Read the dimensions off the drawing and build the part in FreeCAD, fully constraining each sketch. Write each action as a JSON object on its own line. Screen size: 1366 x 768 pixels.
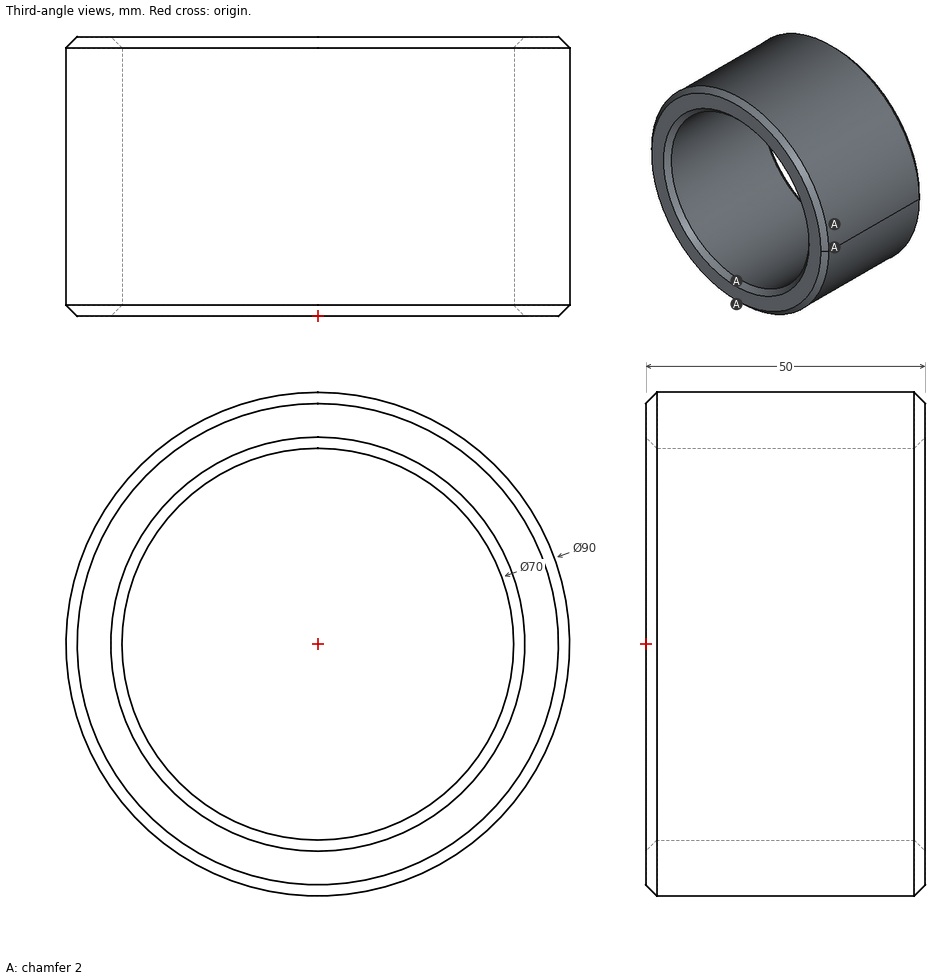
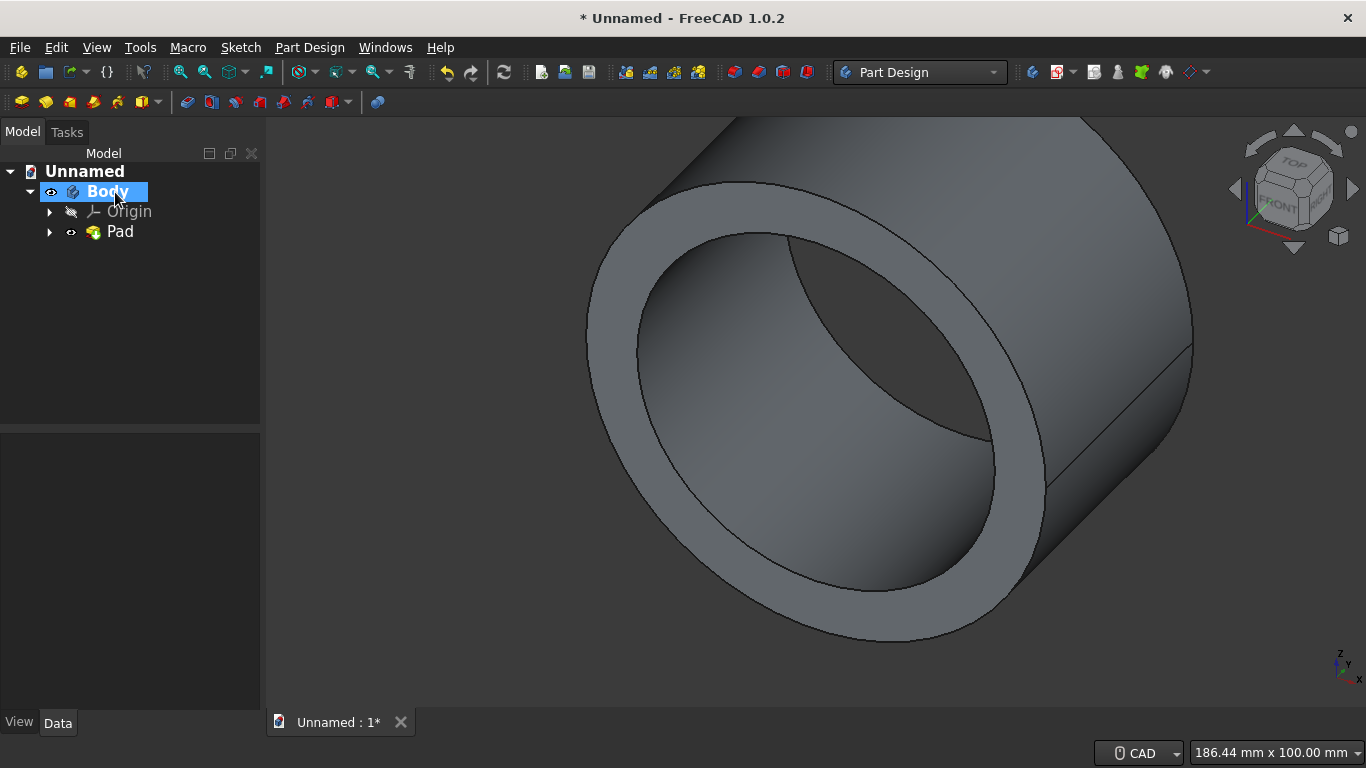
{"action": "left_click", "coordinate": [182, 72]}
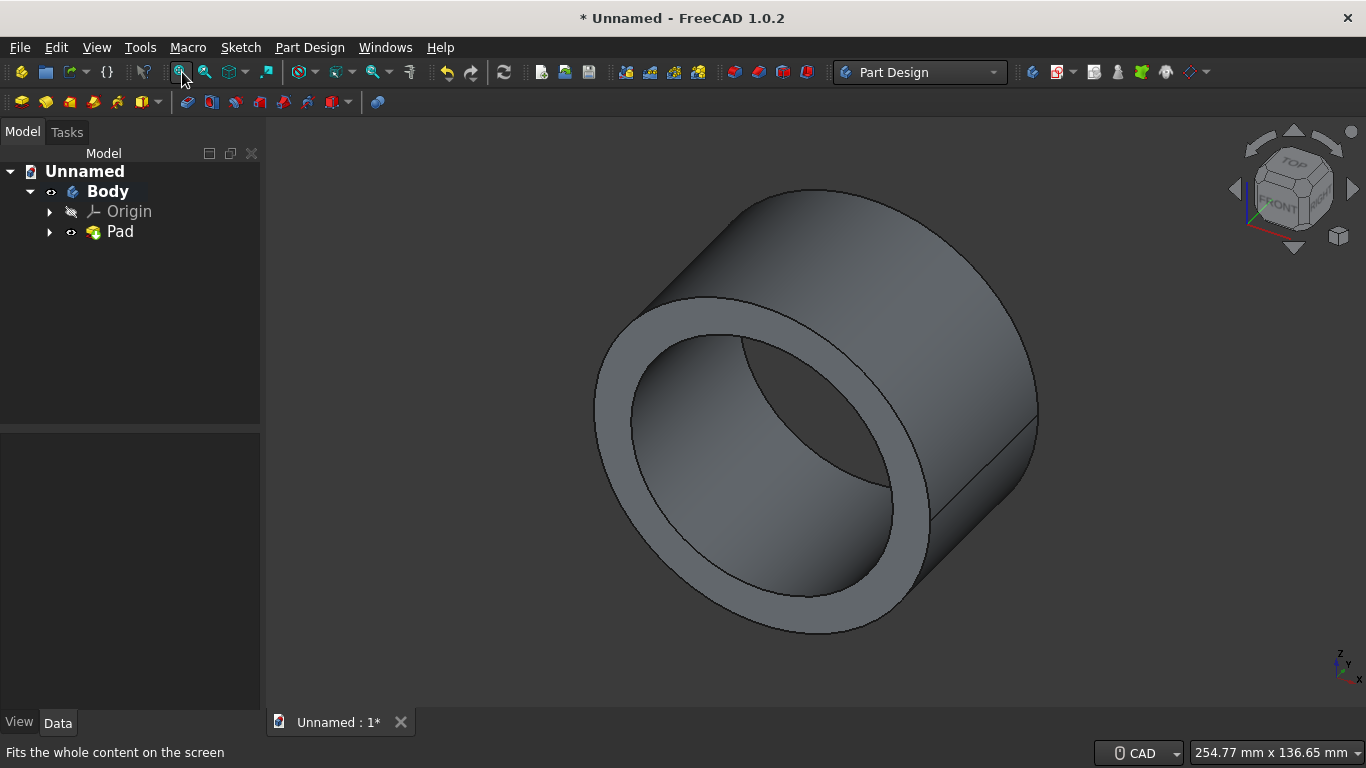
{"action": "left_click", "coordinate": [626, 326]}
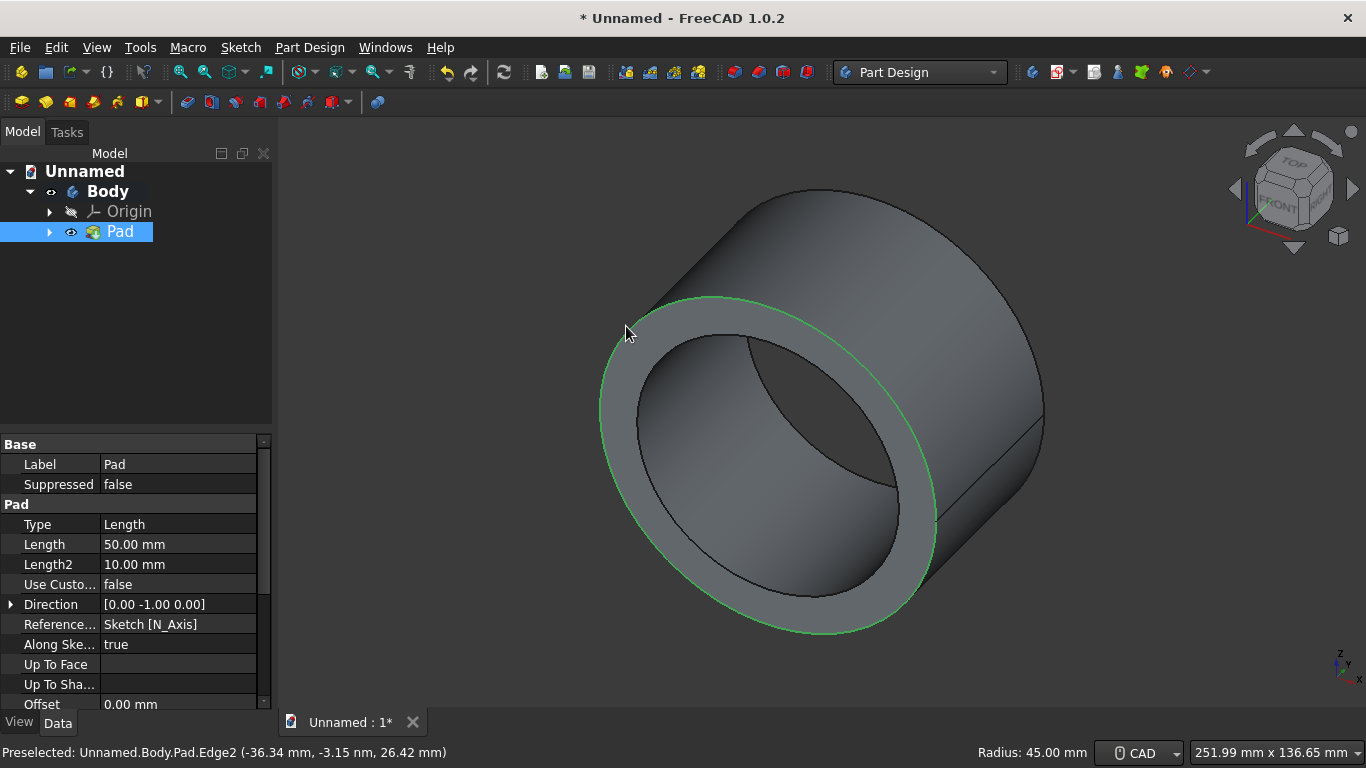
{"action": "left_click", "coordinate": [637, 421], "text": "ctrl"}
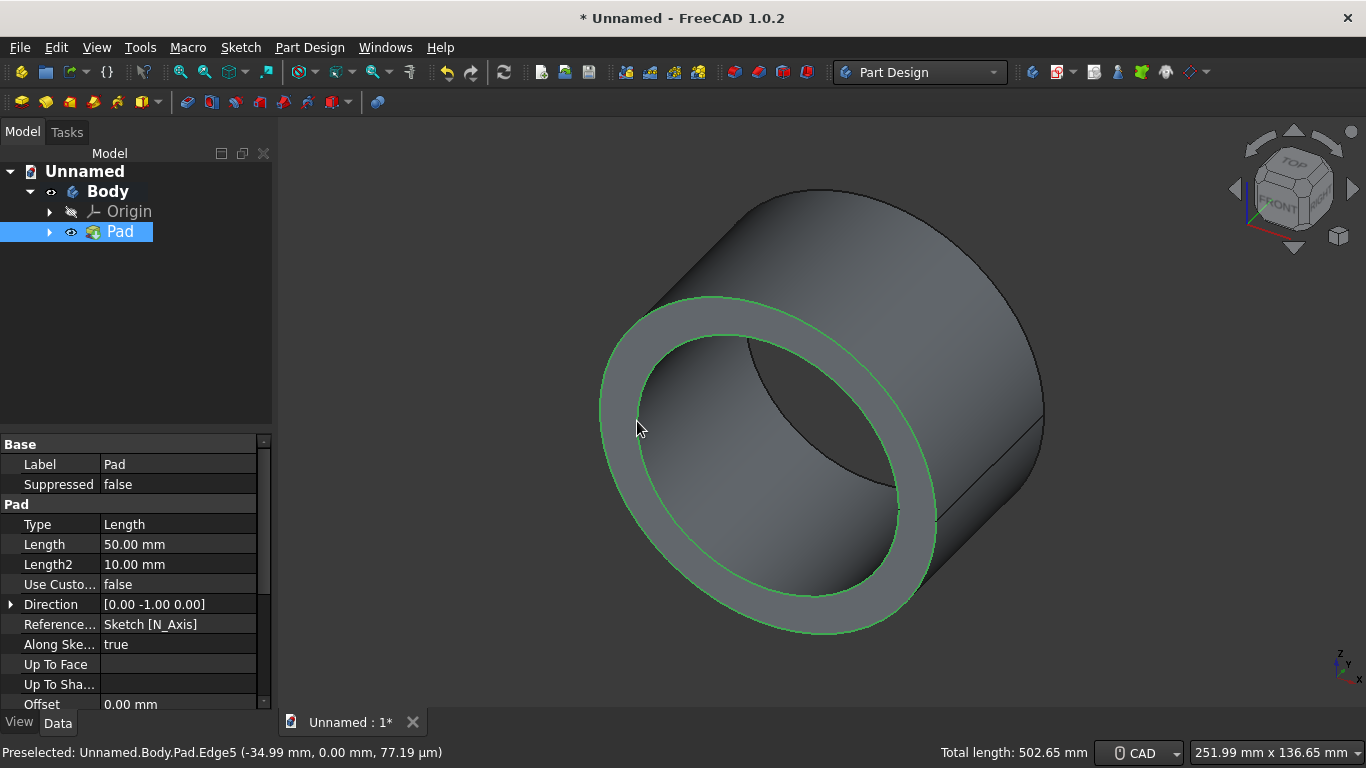
{"action": "key", "text": "0"}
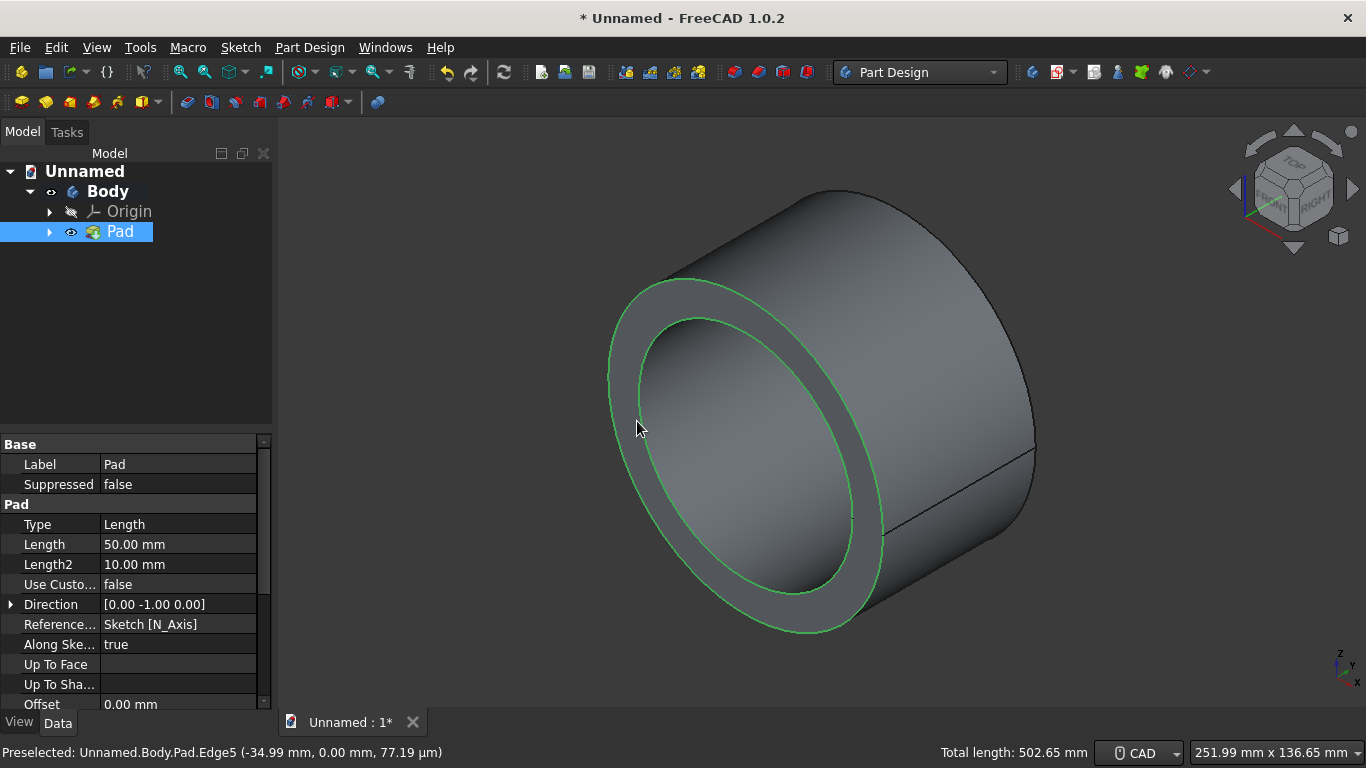
{"action": "key", "text": "2"}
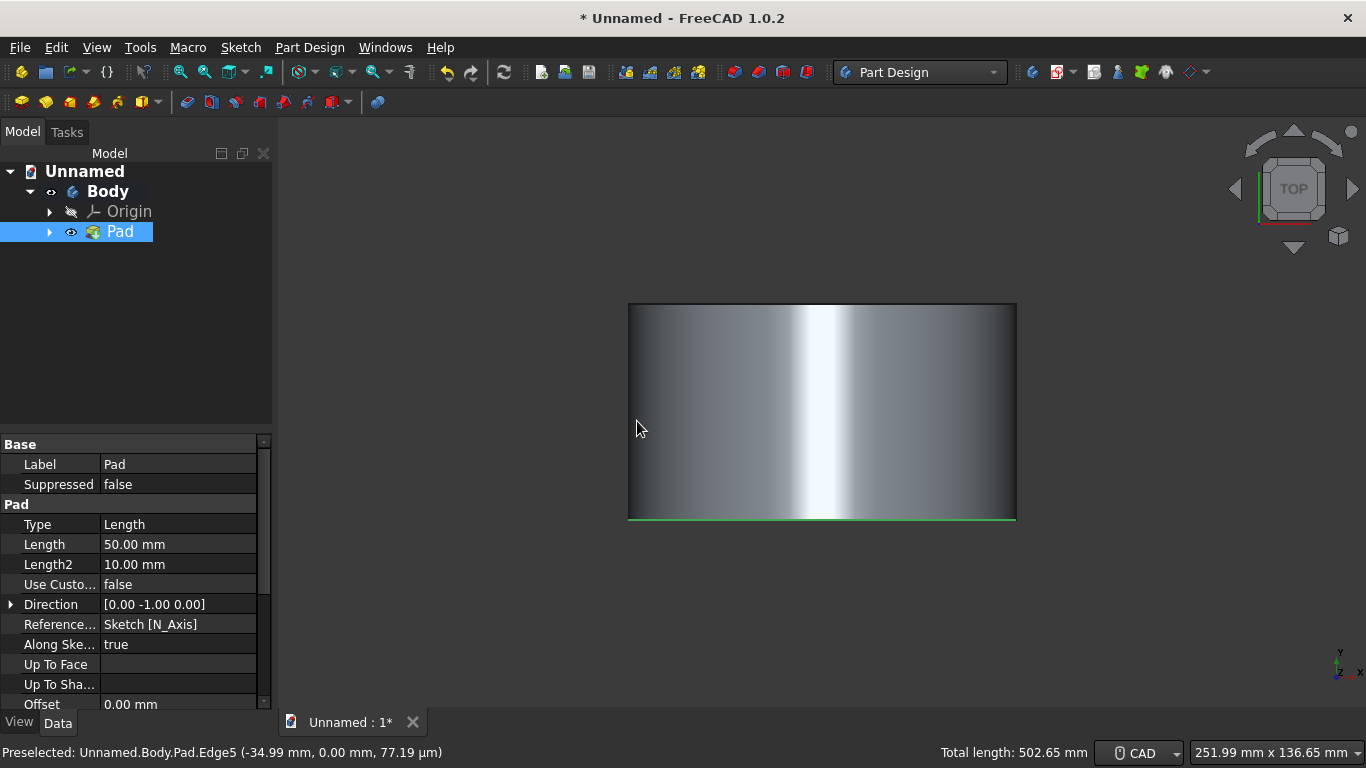
{"action": "left_click", "coordinate": [182, 72]}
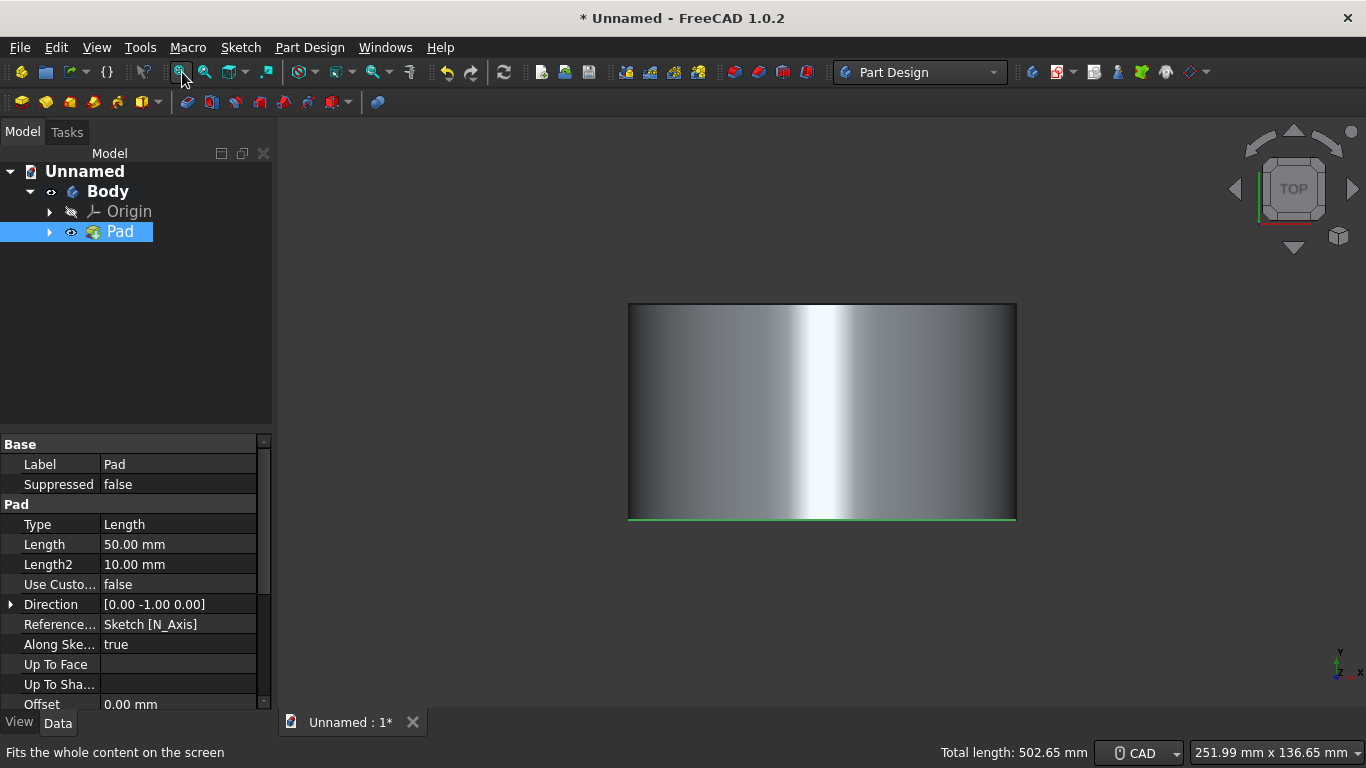
{"action": "left_click", "coordinate": [665, 303], "text": "ctrl"}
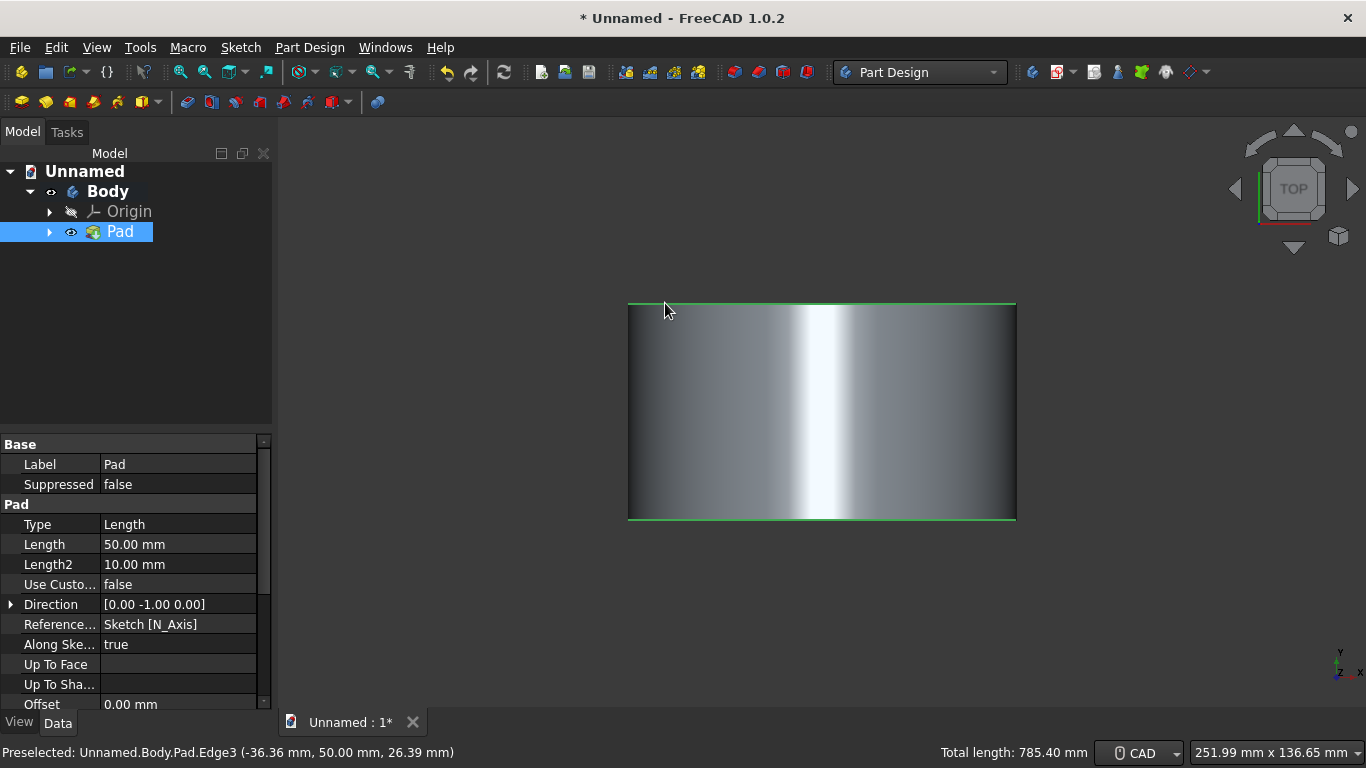
{"action": "key", "text": "1"}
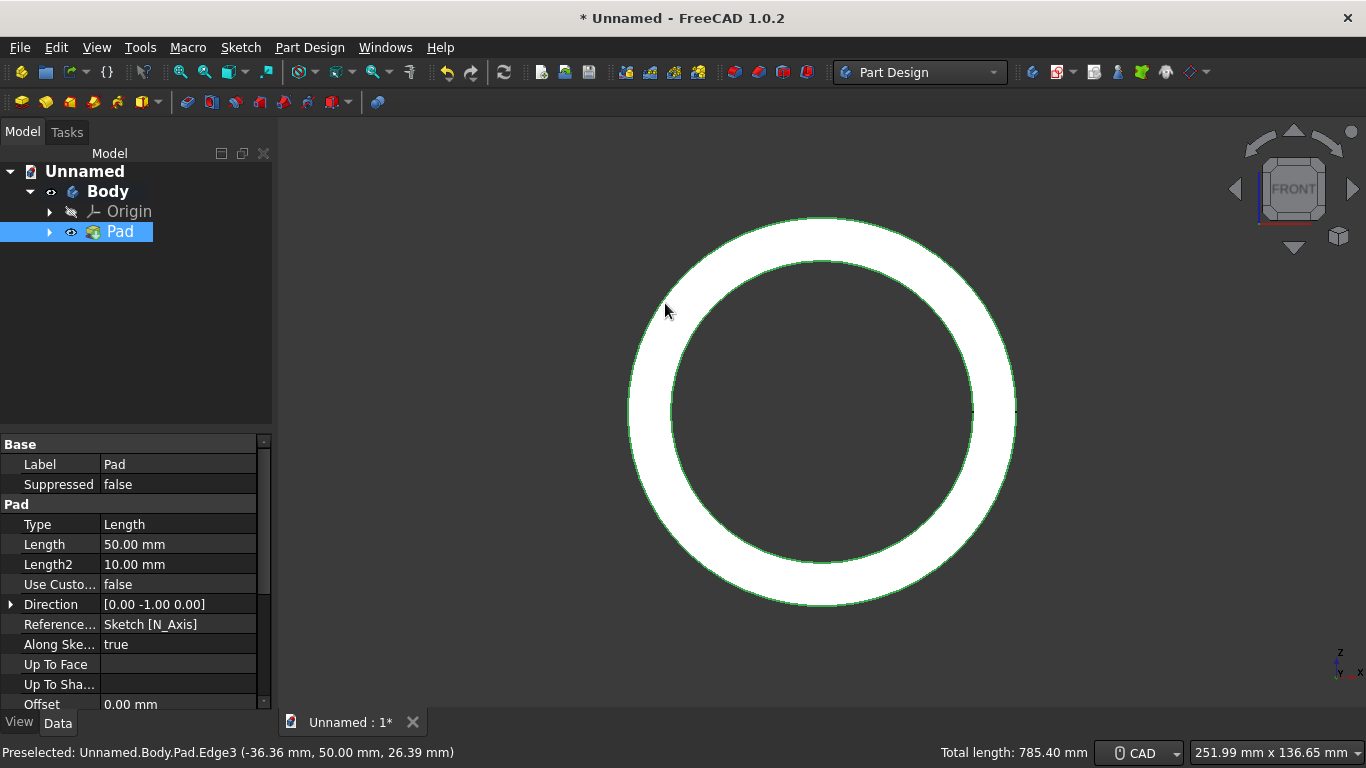
{"action": "key", "text": "3"}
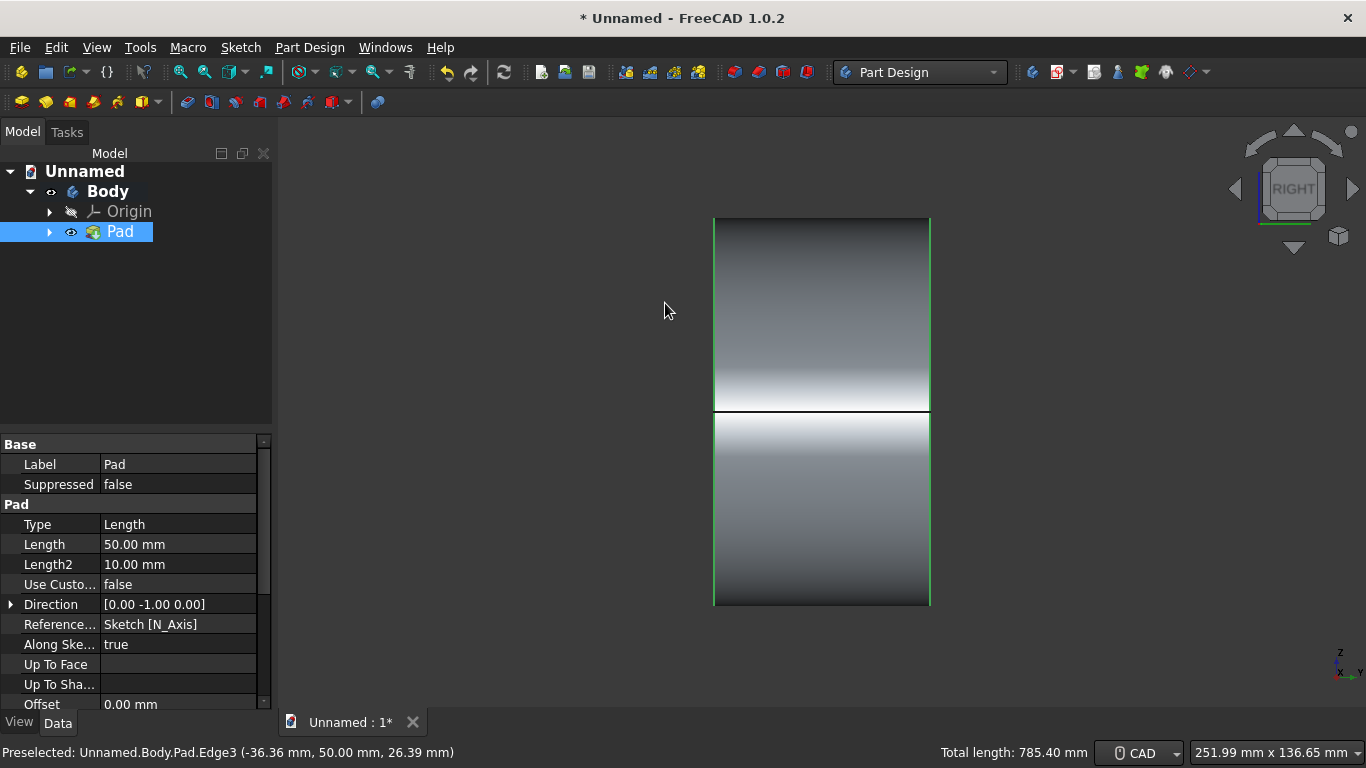
{"action": "key", "text": "5"}